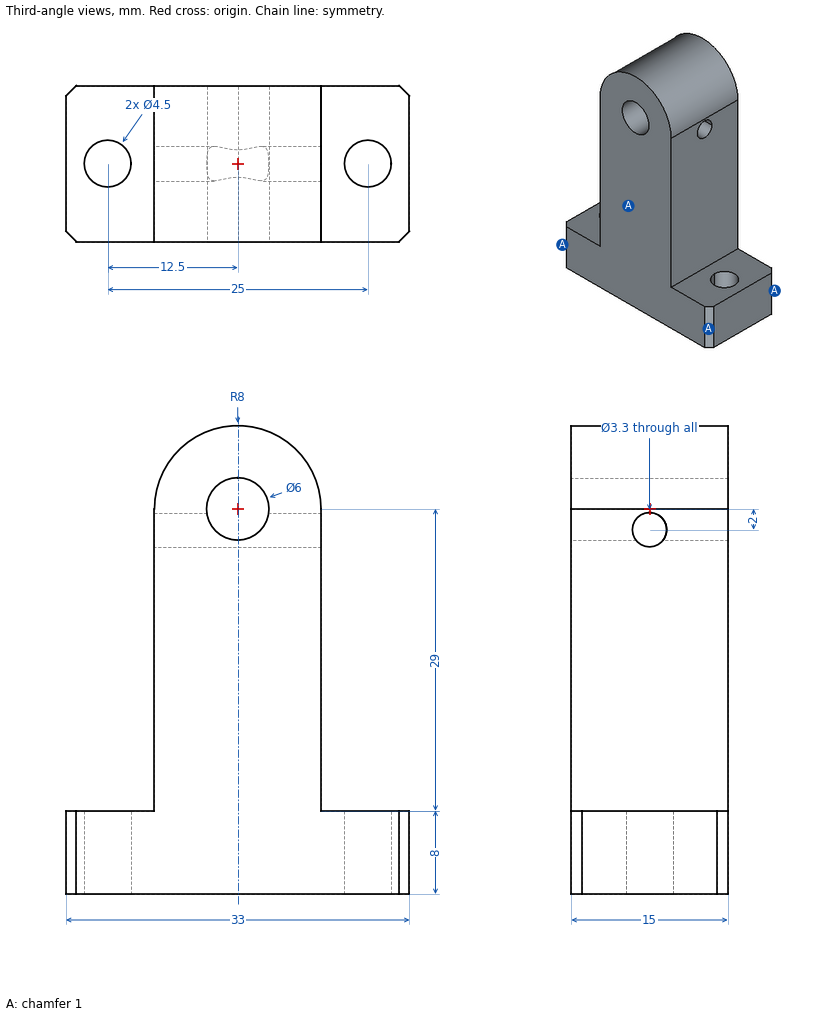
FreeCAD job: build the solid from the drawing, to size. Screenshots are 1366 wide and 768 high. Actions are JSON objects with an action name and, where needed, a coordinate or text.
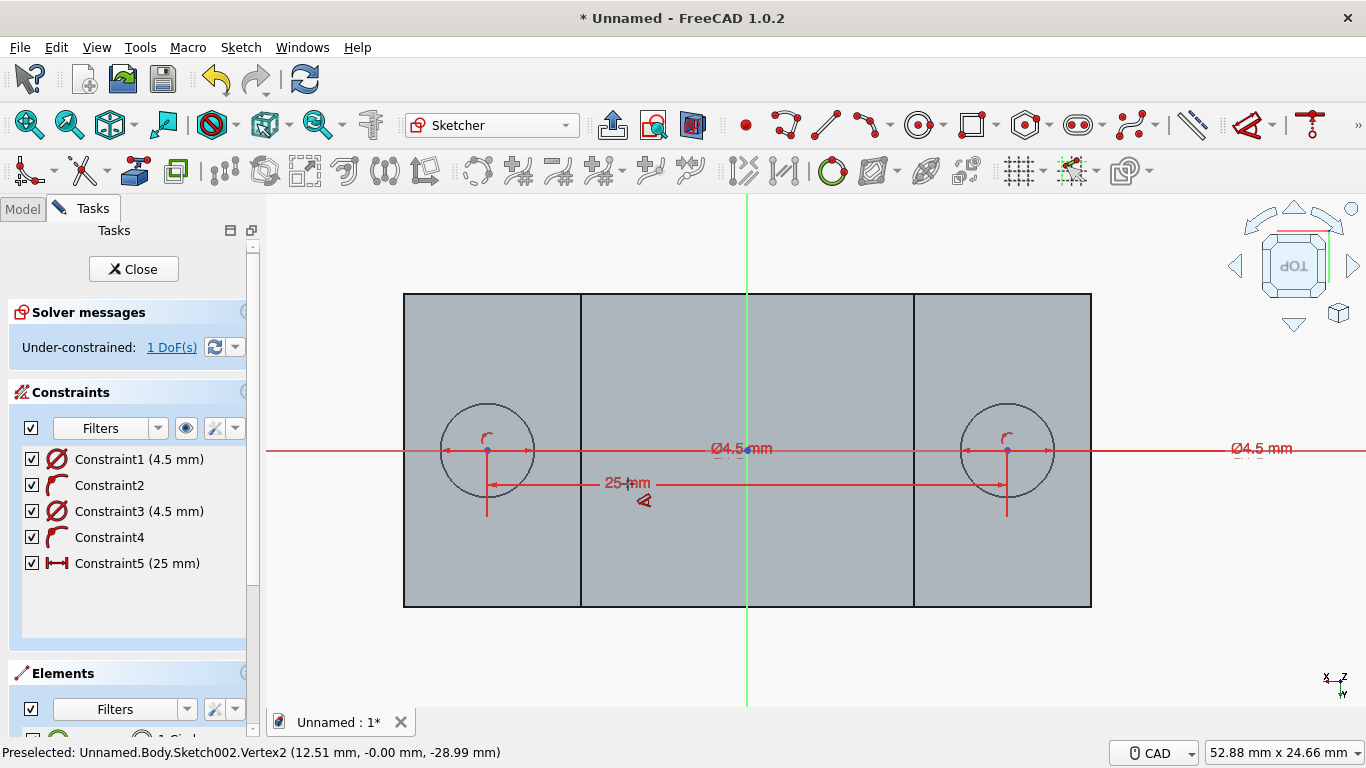
{"action": "left_click", "coordinate": [1007, 450]}
{"action": "left_click", "coordinate": [877, 484]}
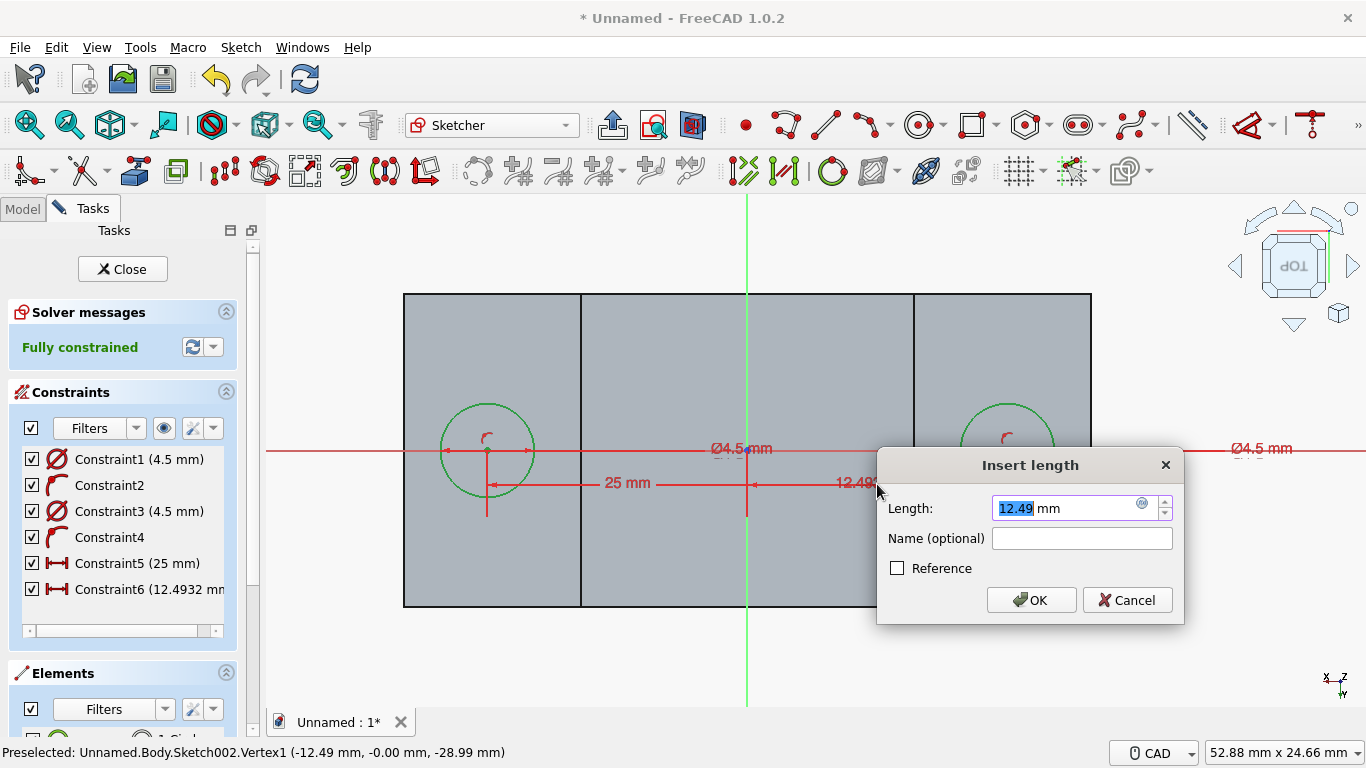
{"action": "type", "text": "12.5"}
{"action": "key", "text": "Return"}
{"action": "key", "text": "Escape"}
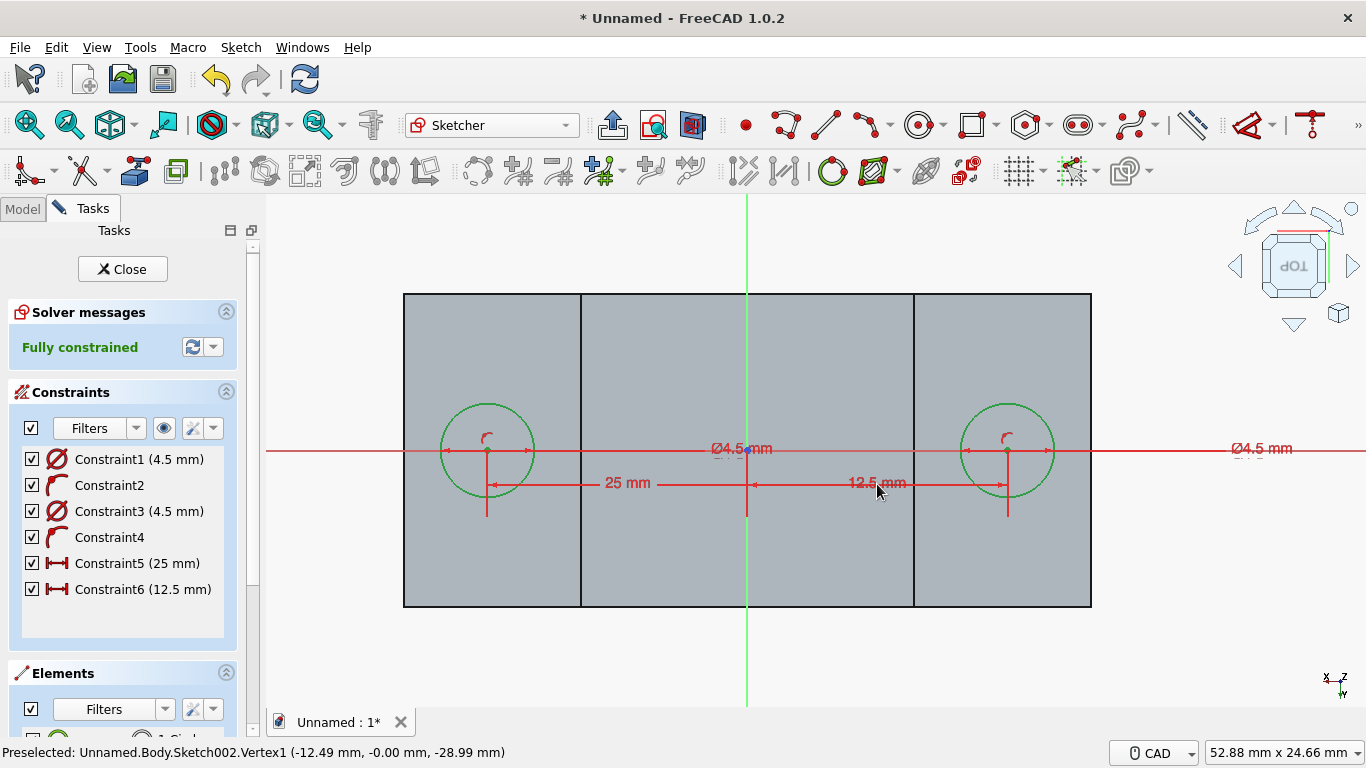
{"action": "left_click", "coordinate": [123, 269]}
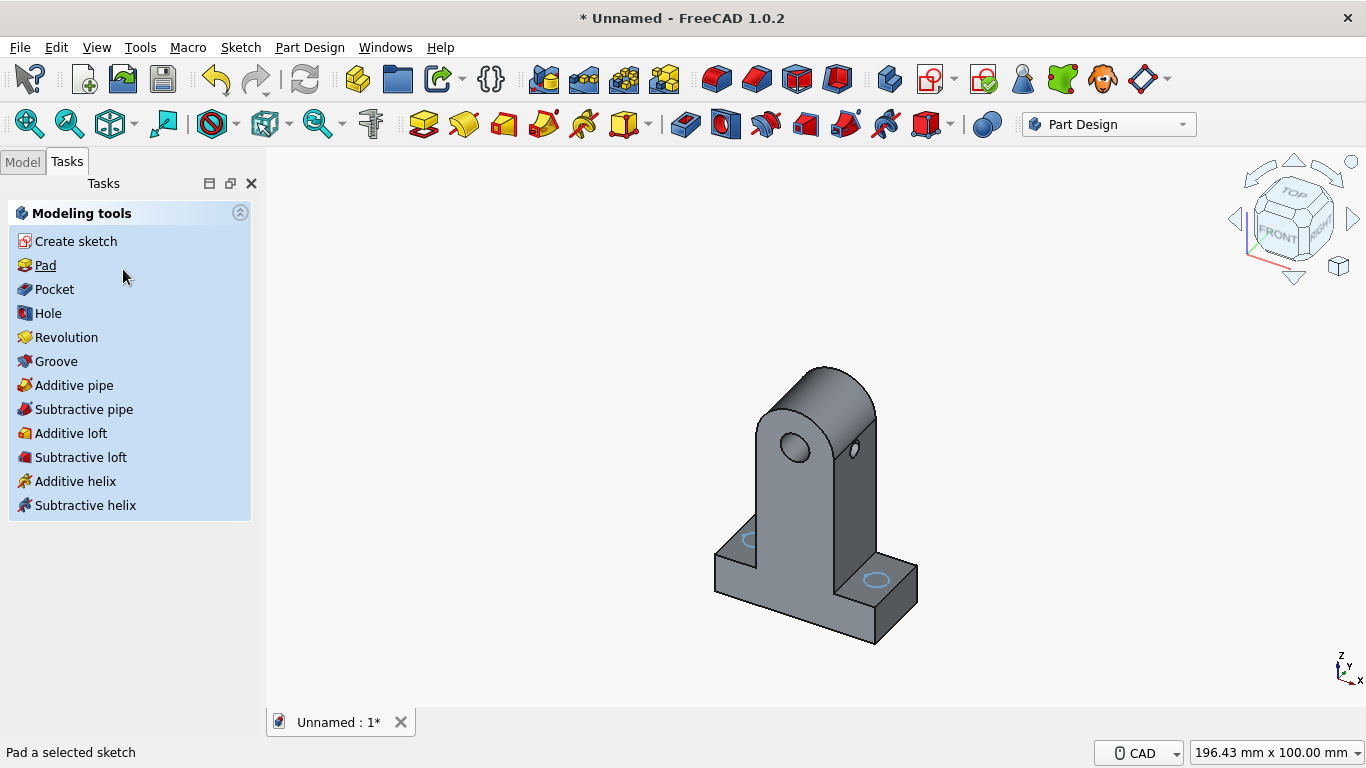
{"action": "left_click", "coordinate": [686, 124]}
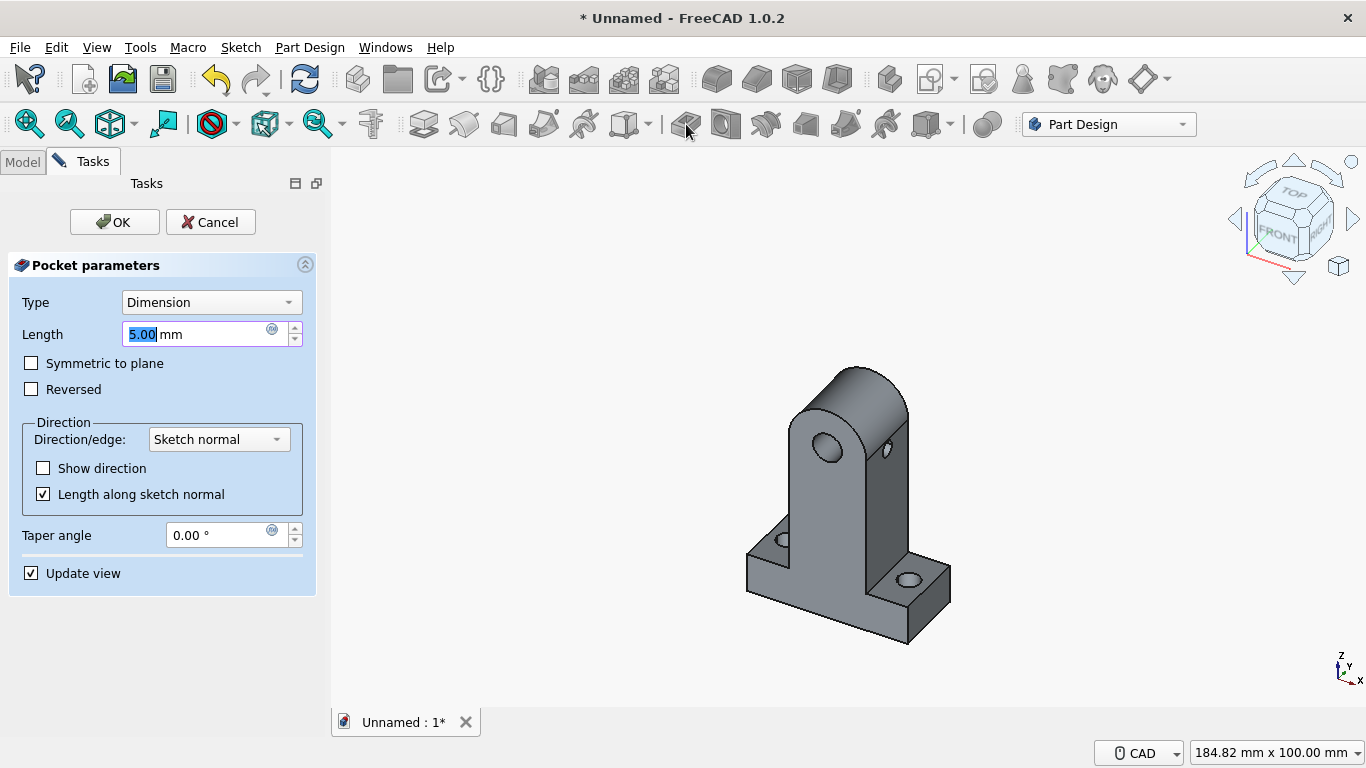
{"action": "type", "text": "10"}
{"action": "key", "text": "Tab"}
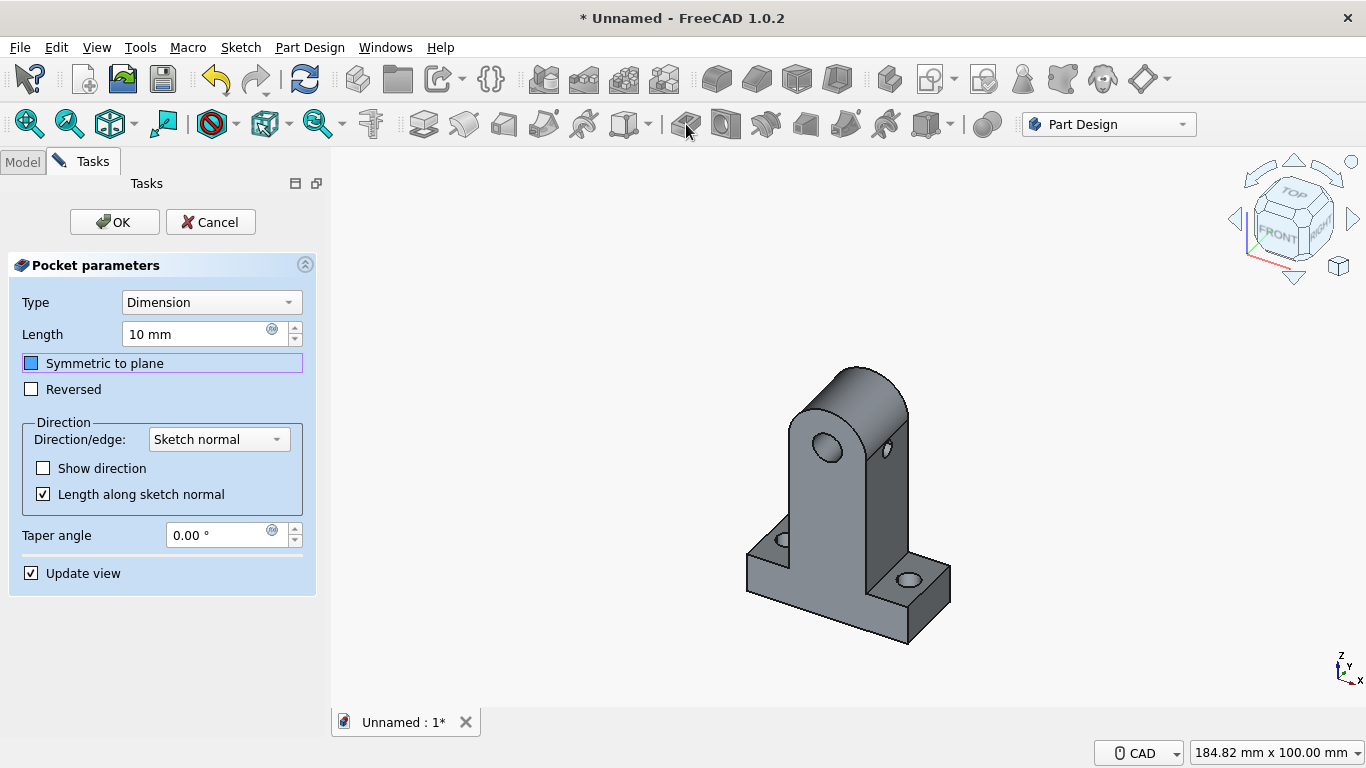
{"action": "left_click", "coordinate": [115, 222]}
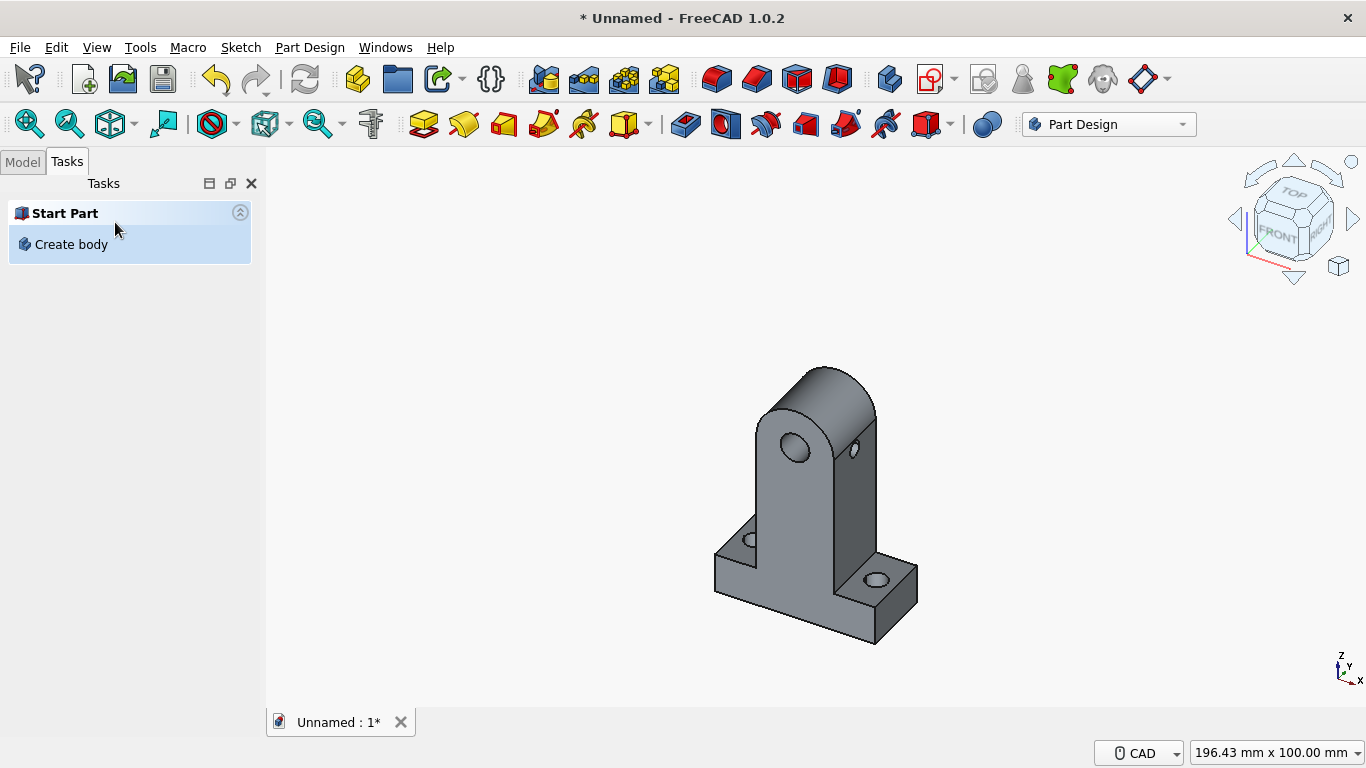
{"action": "left_click", "coordinate": [875, 625]}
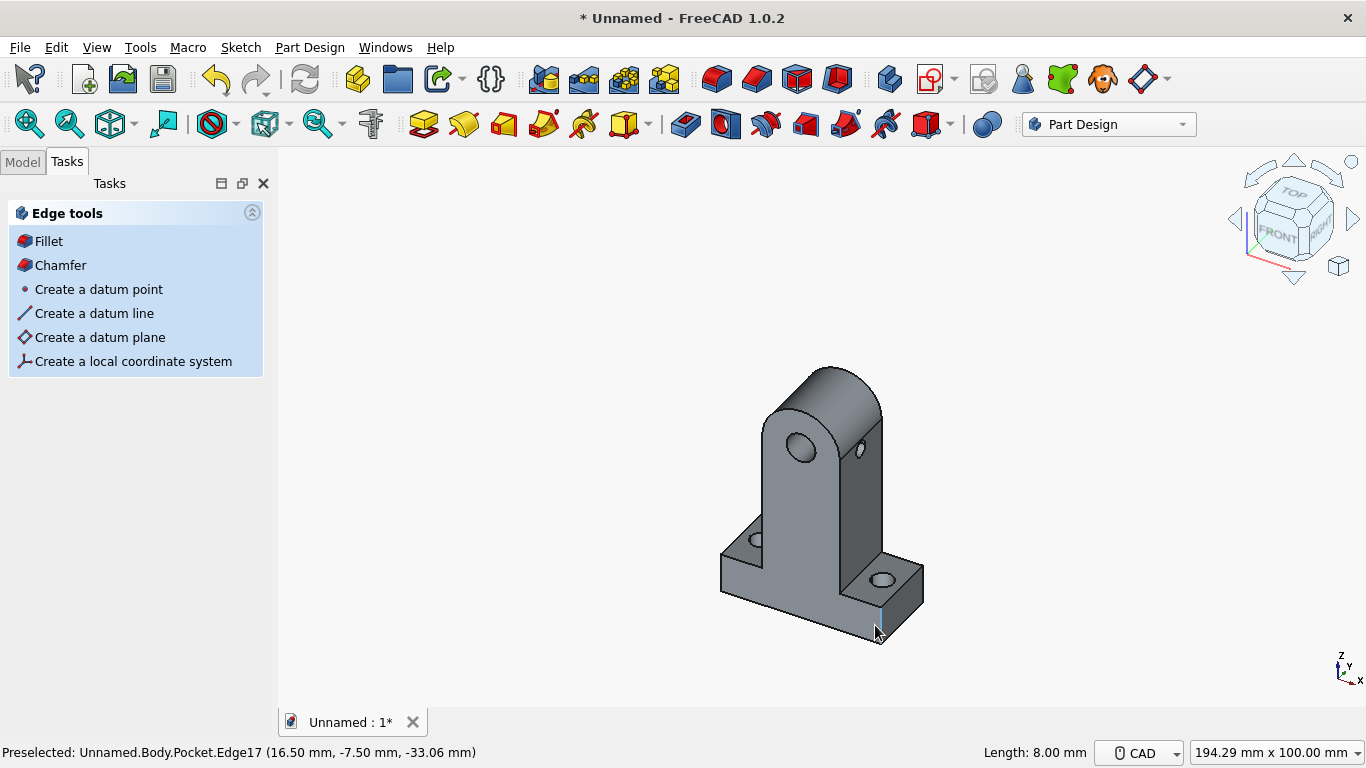
{"action": "key", "text": "0"}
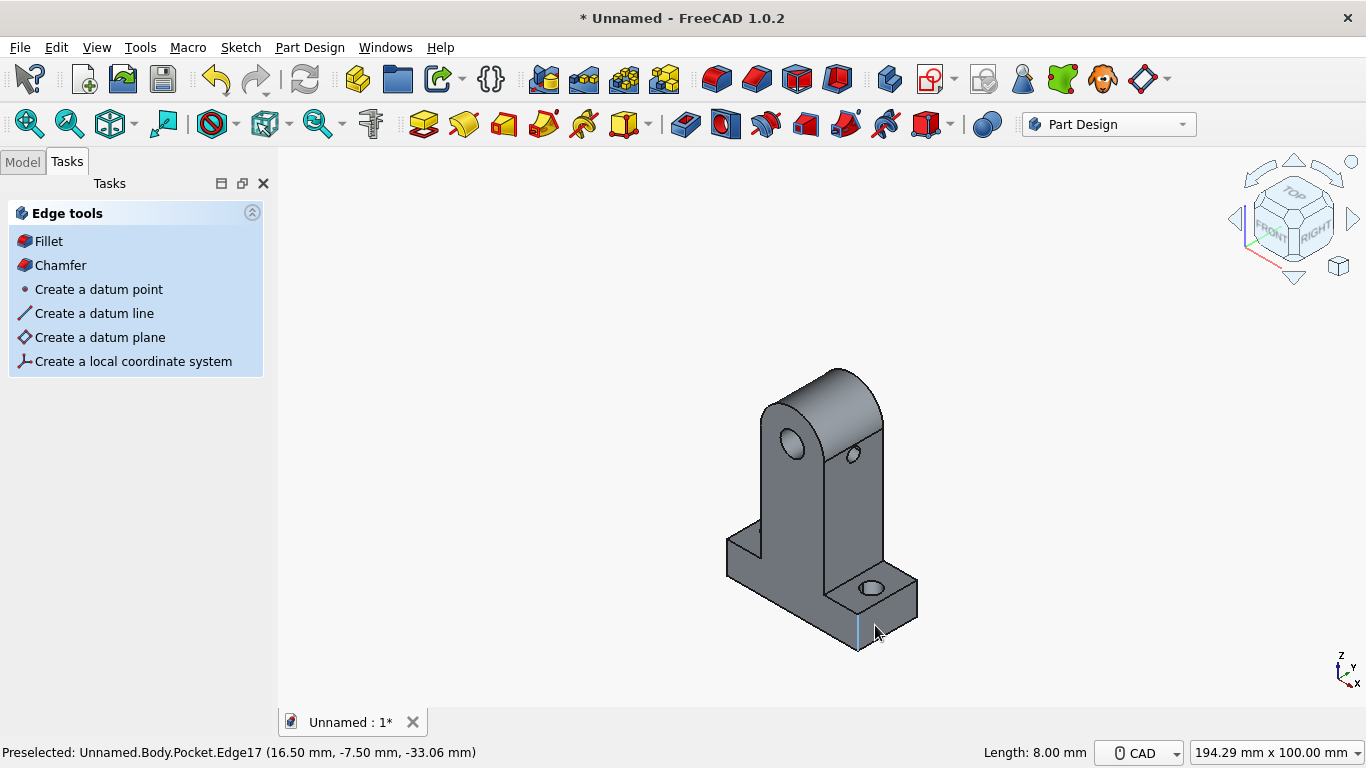
{"action": "key", "text": "2"}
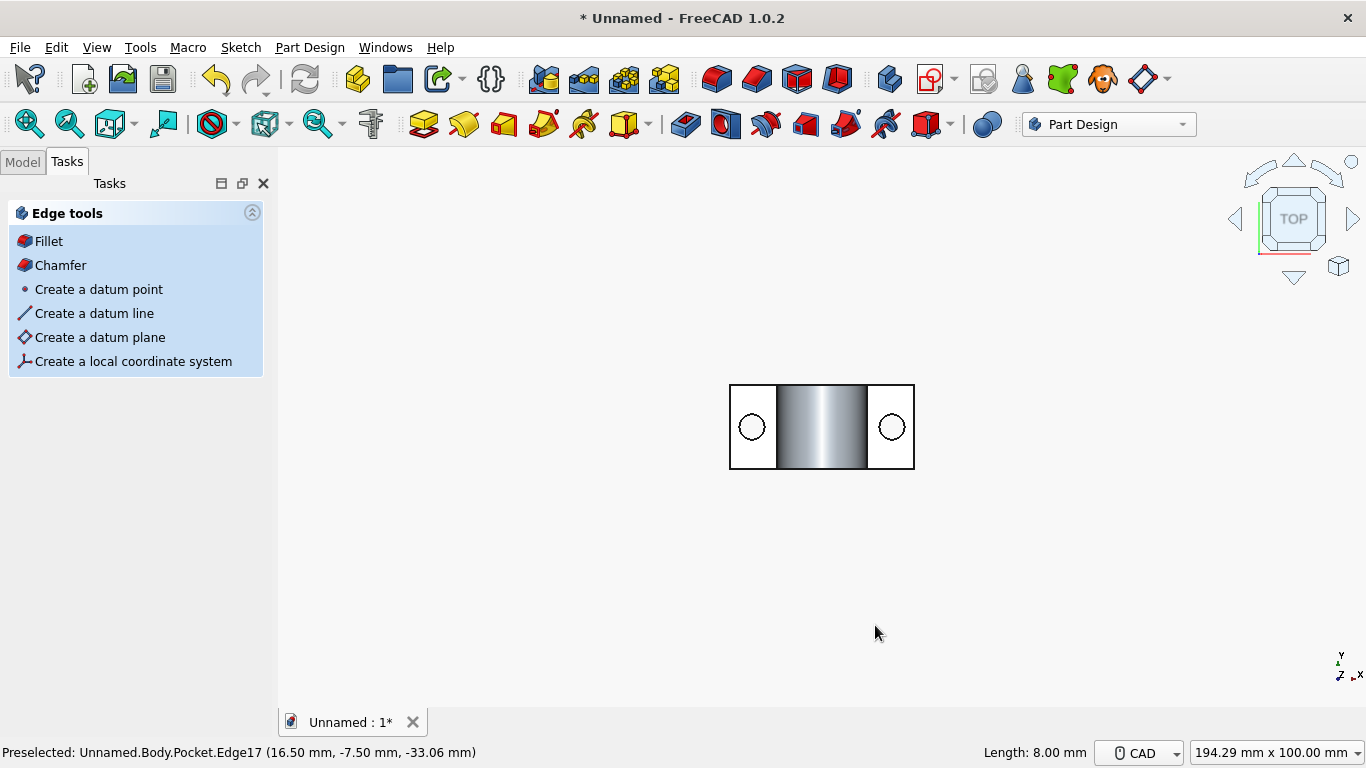
{"action": "key", "text": "v f"}